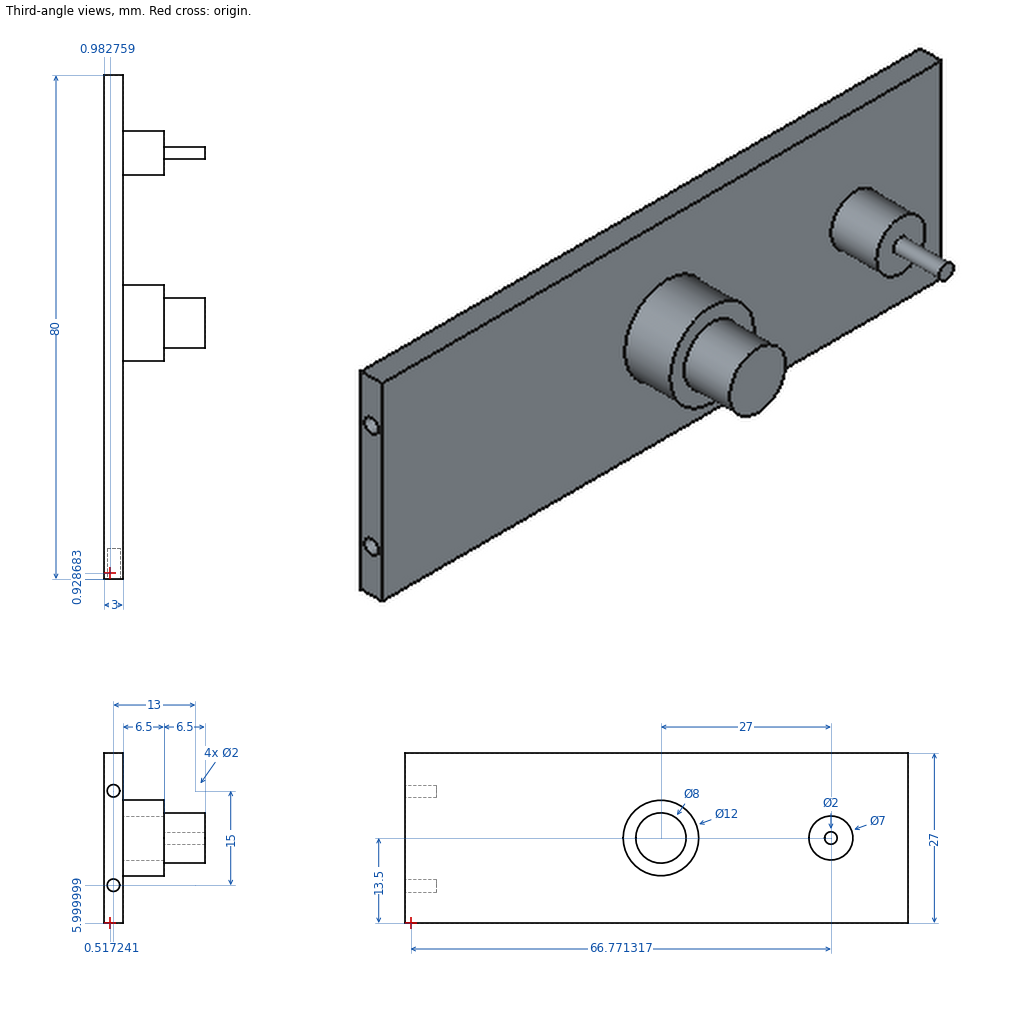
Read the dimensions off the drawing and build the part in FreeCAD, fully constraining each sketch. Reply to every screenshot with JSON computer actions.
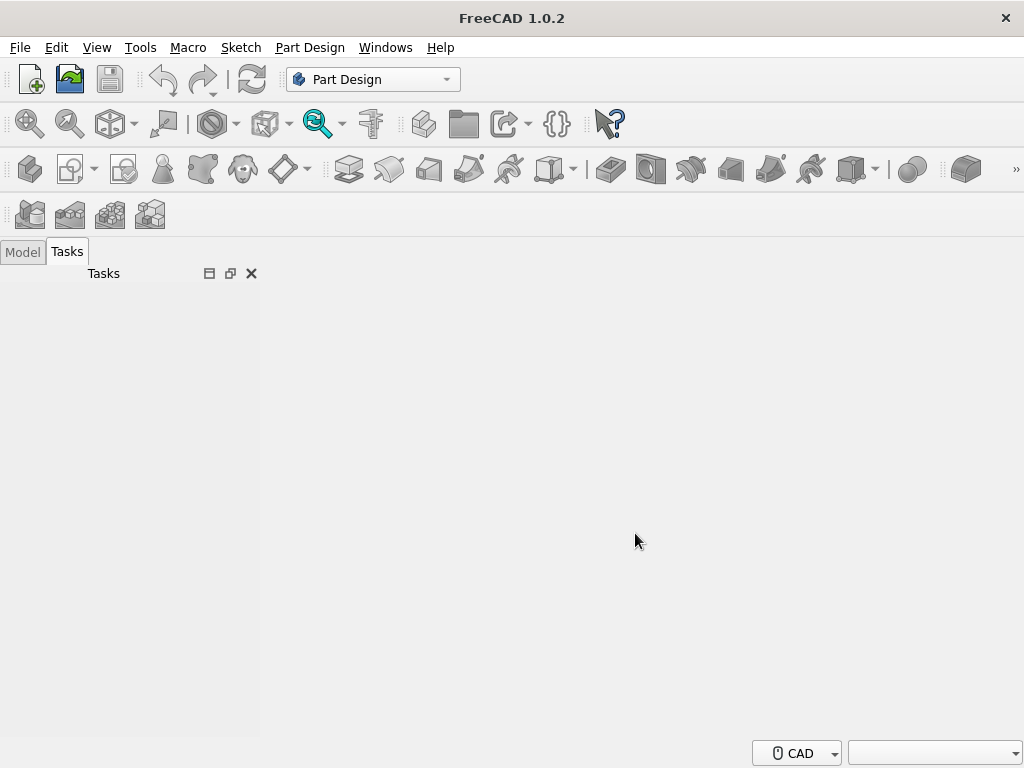
{"action": "left_click", "coordinate": [30, 80]}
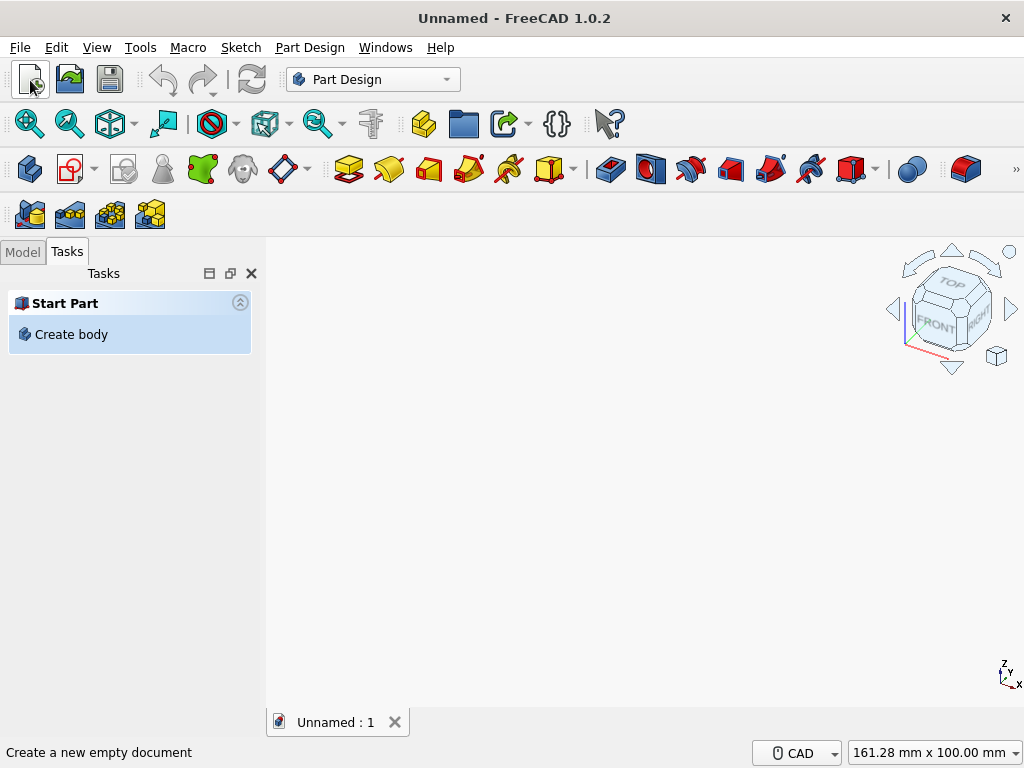
{"action": "left_click", "coordinate": [70, 170]}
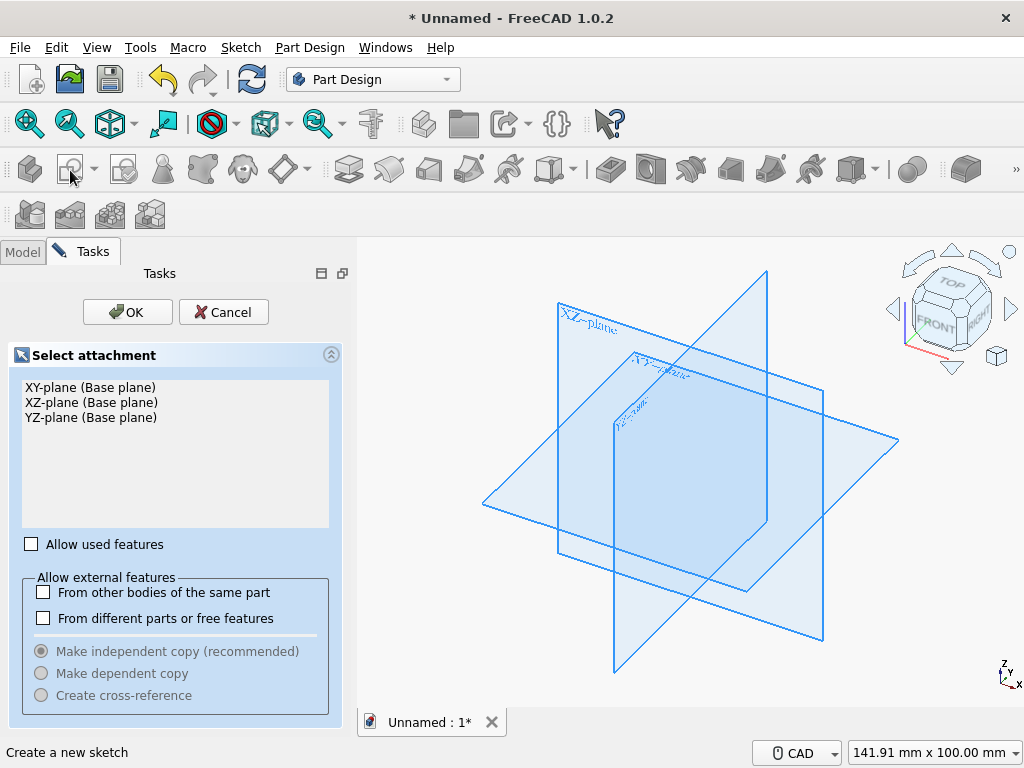
{"action": "left_click", "coordinate": [82, 388]}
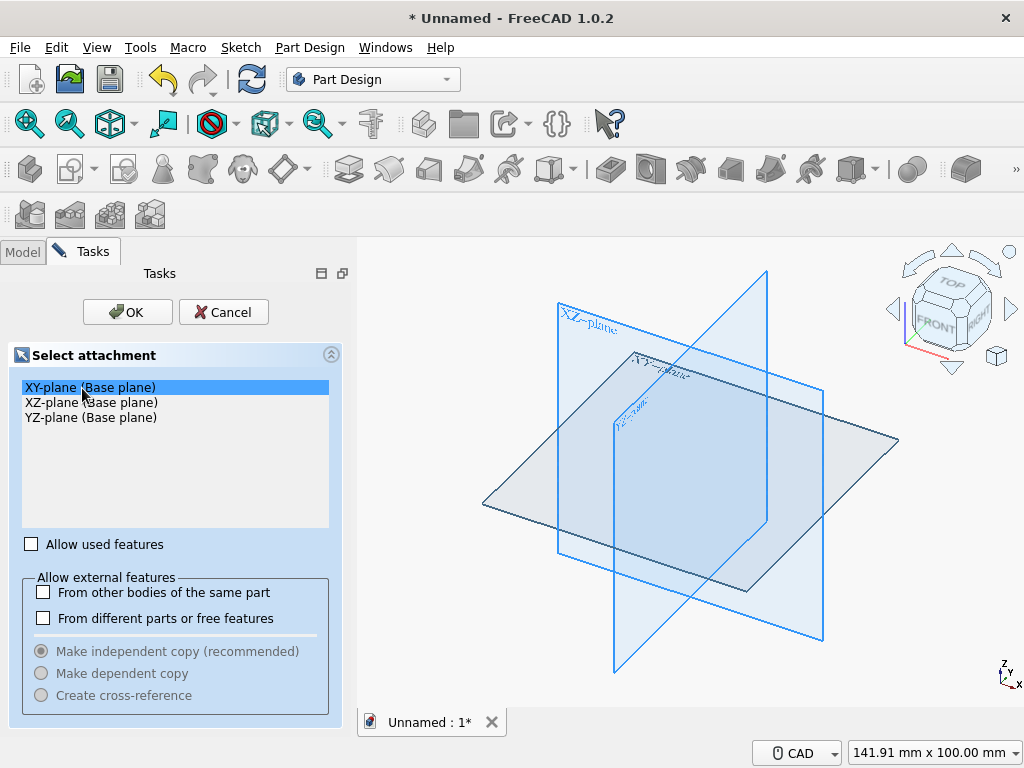
{"action": "left_click", "coordinate": [128, 312]}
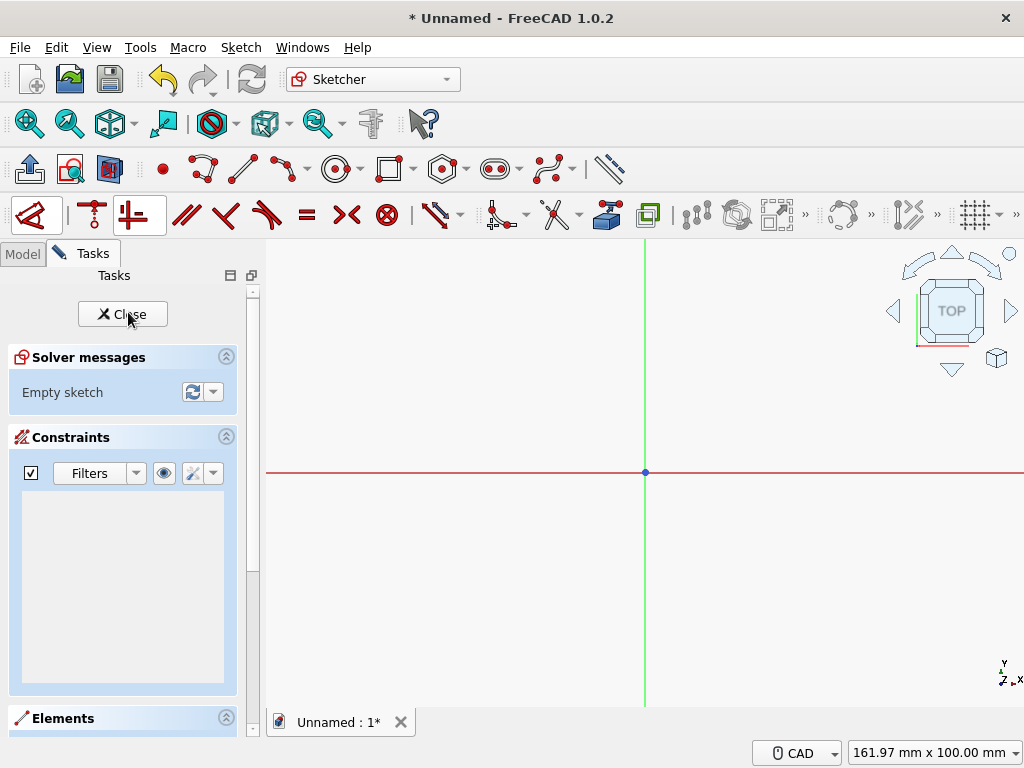
{"action": "scroll", "coordinate": [432, 679], "scroll_direction": "down", "scroll_amount": 2}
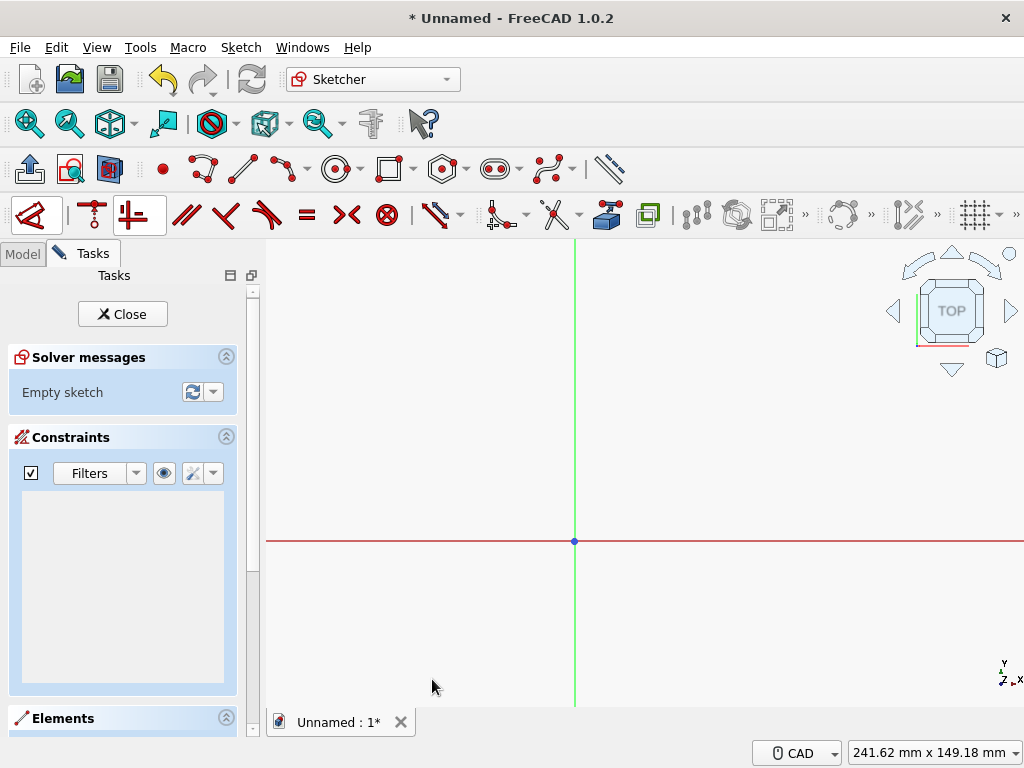
{"action": "left_click", "coordinate": [390, 170]}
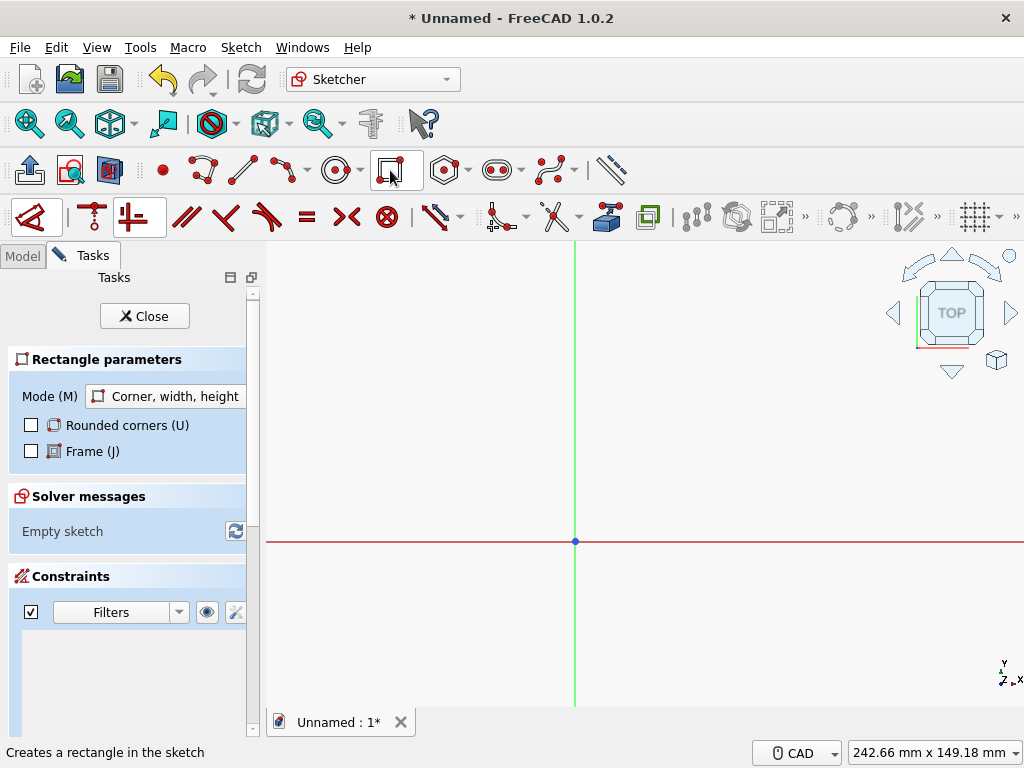
{"action": "scroll", "coordinate": [572, 295], "scroll_direction": "up", "scroll_amount": 9}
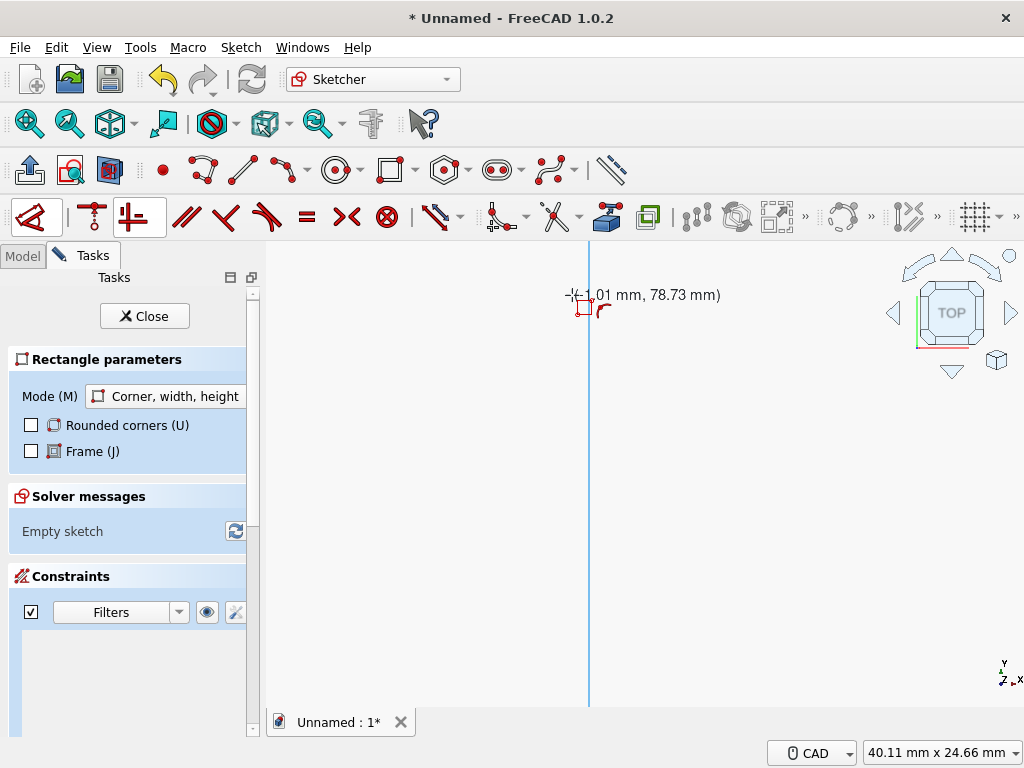
{"action": "left_click", "coordinate": [570, 294]}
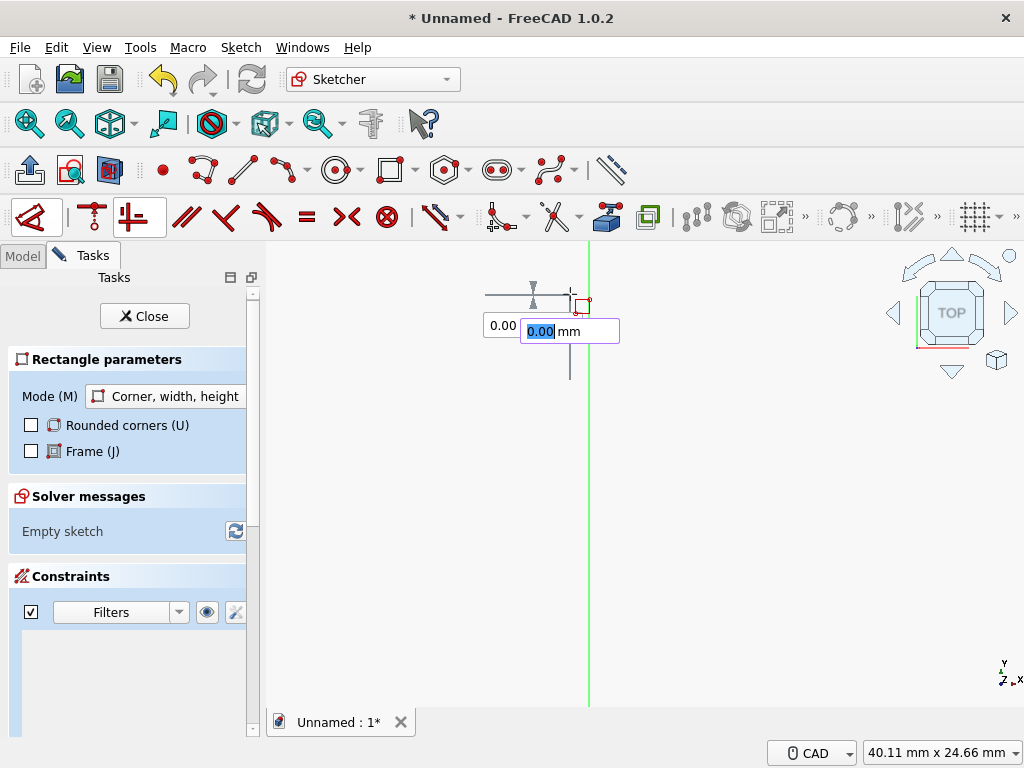
{"action": "scroll", "coordinate": [571, 328], "scroll_direction": "down", "scroll_amount": 8}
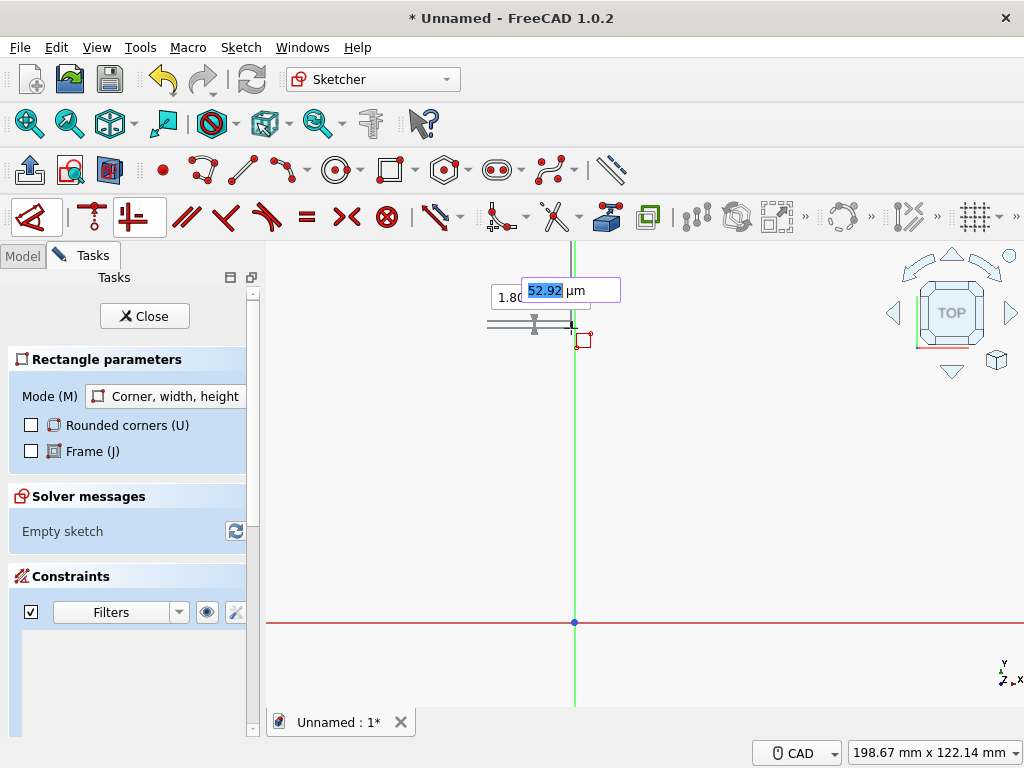
{"action": "scroll", "coordinate": [583, 627], "scroll_direction": "up", "scroll_amount": 8}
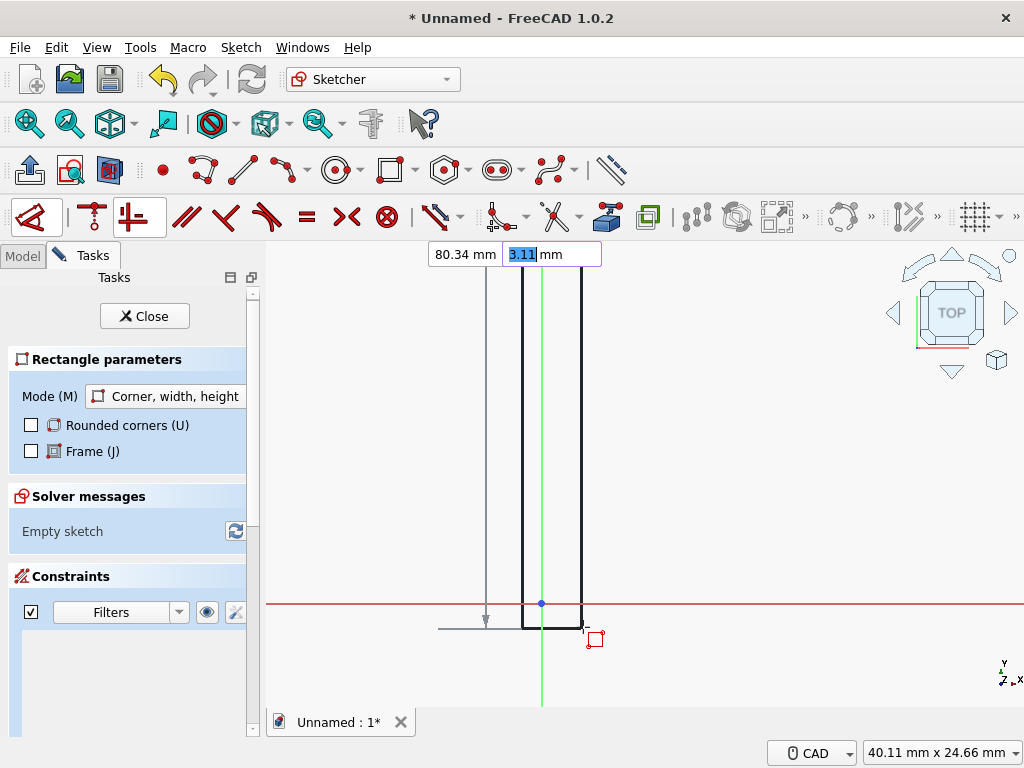
{"action": "left_click", "coordinate": [580, 621]}
{"action": "key", "text": "Escape"}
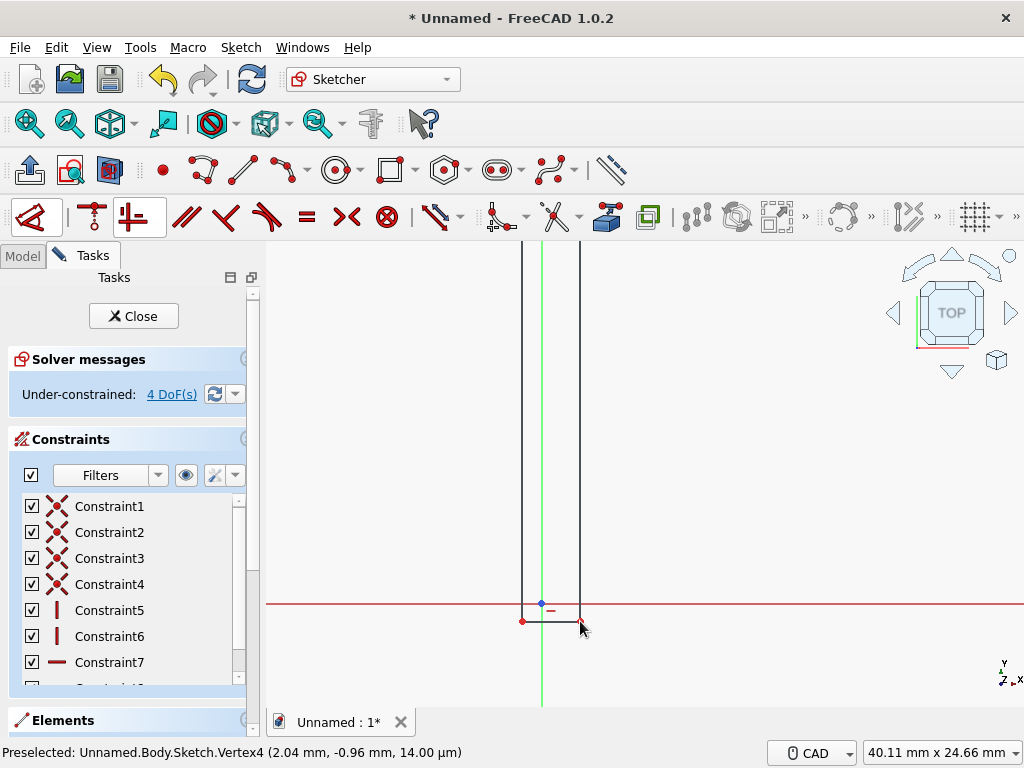
{"action": "left_click", "coordinate": [540, 622]}